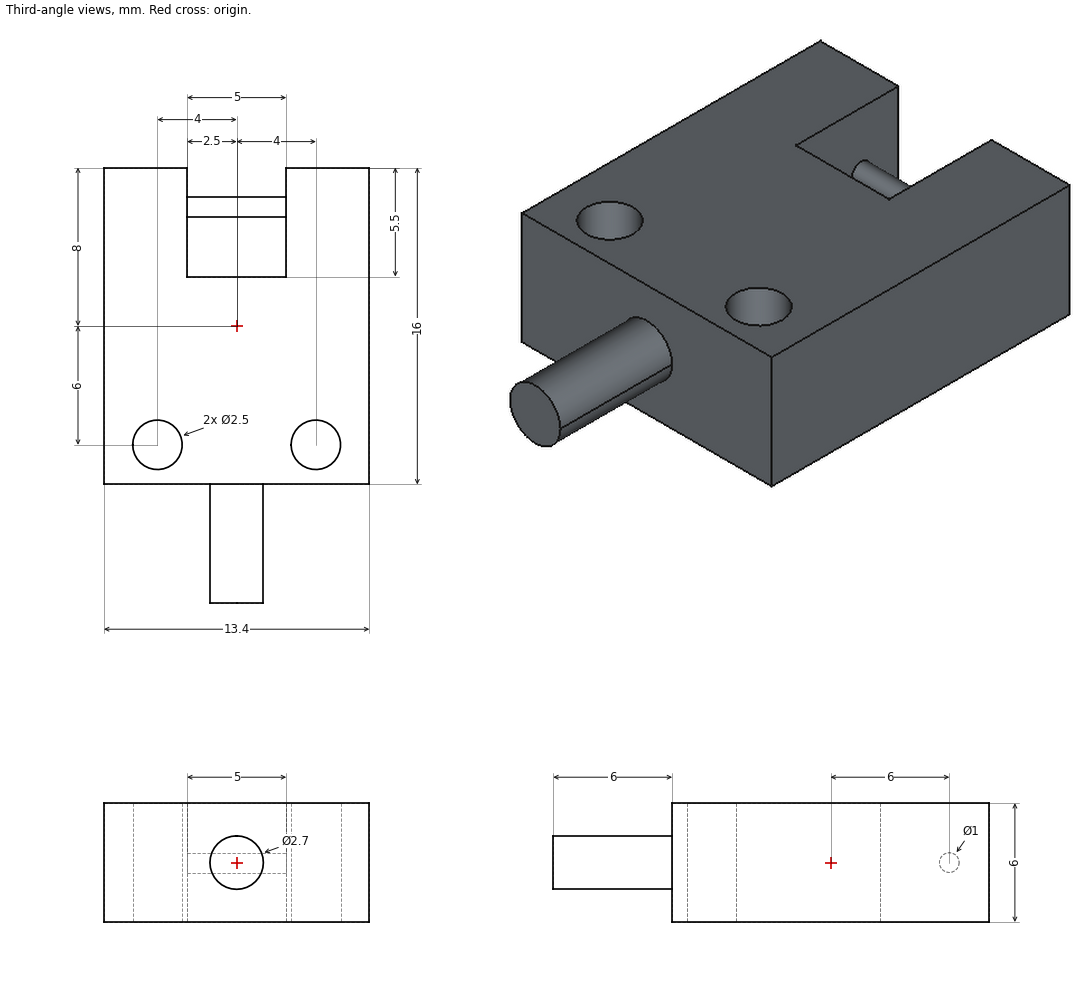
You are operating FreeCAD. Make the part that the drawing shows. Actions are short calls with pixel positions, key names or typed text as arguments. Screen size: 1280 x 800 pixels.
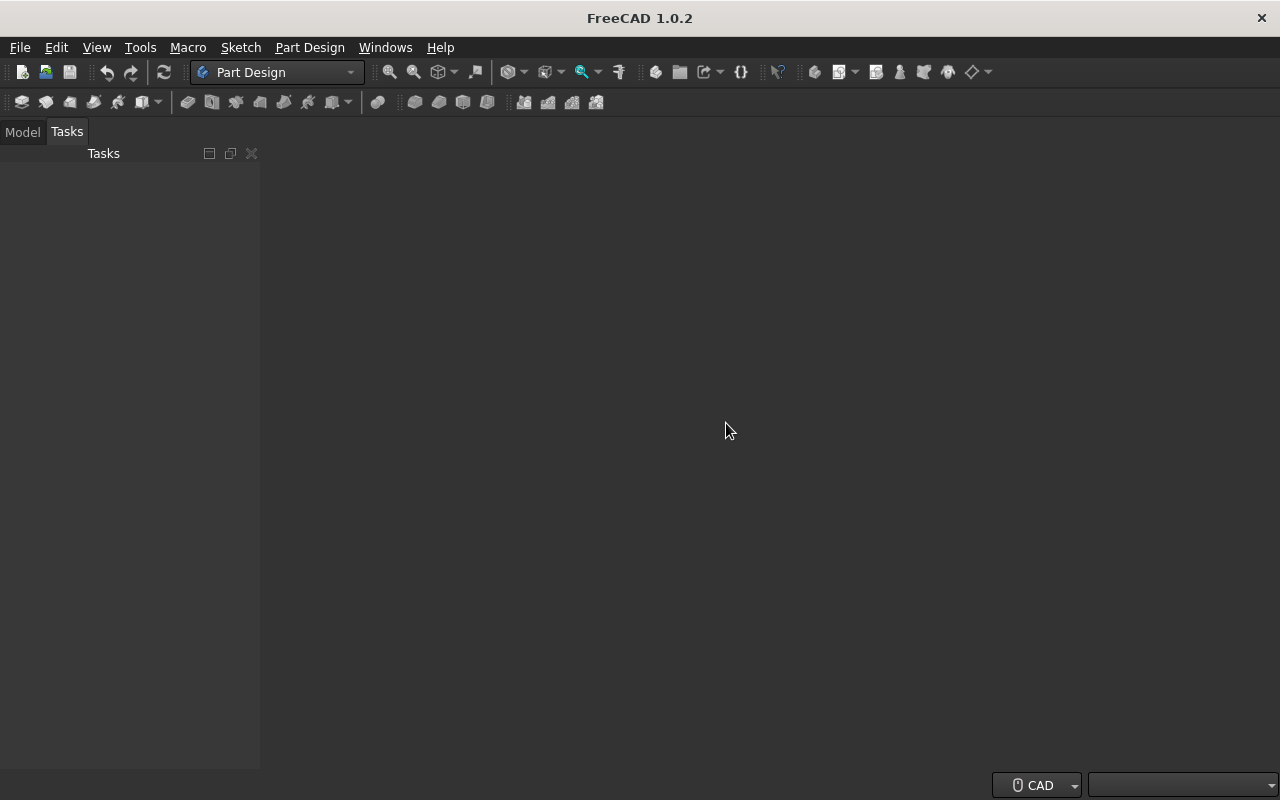
click(22, 72)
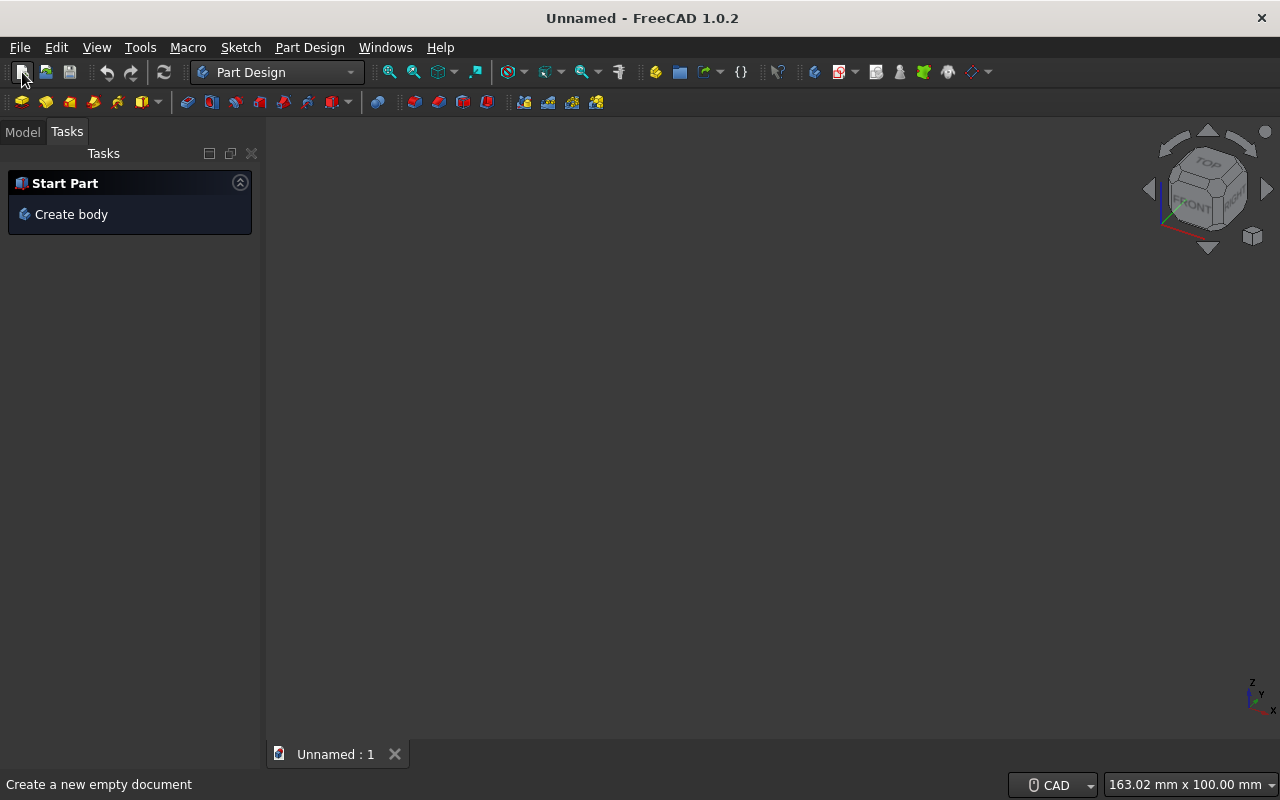
click(840, 72)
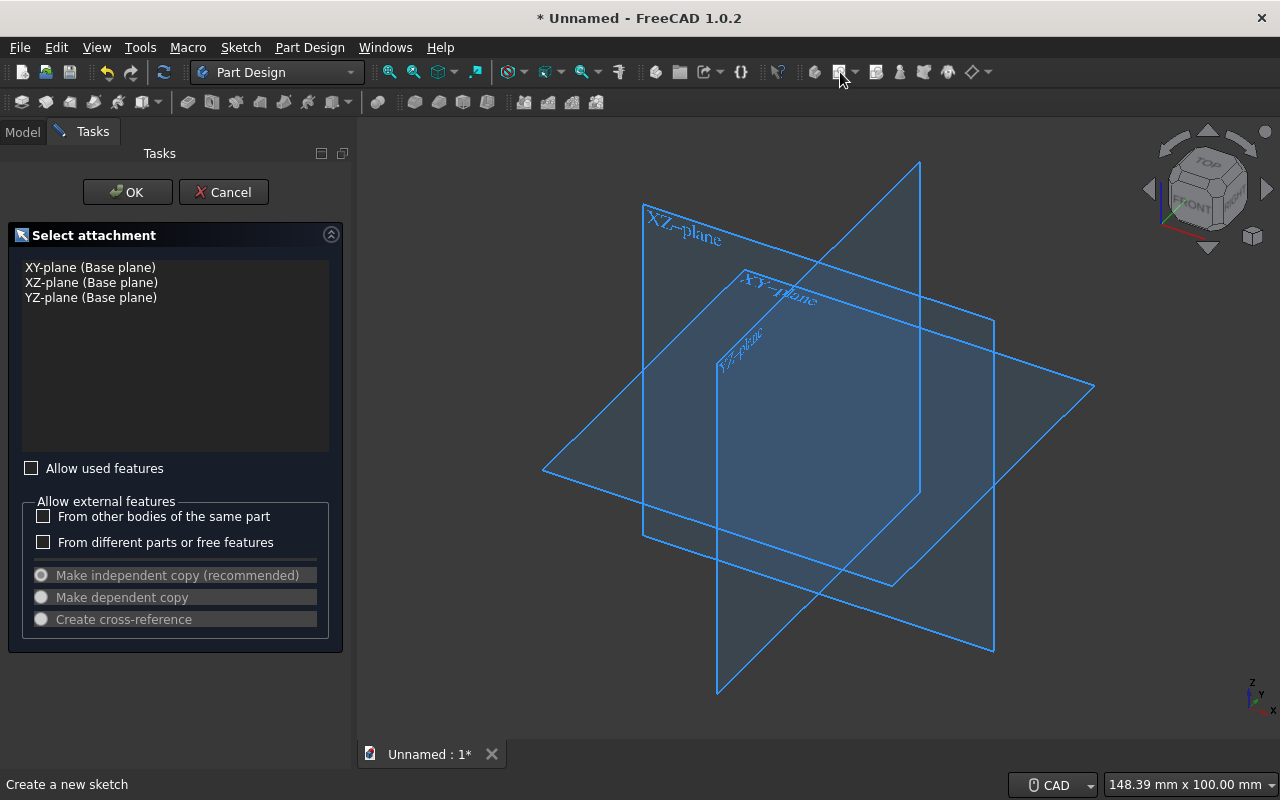
click(82, 268)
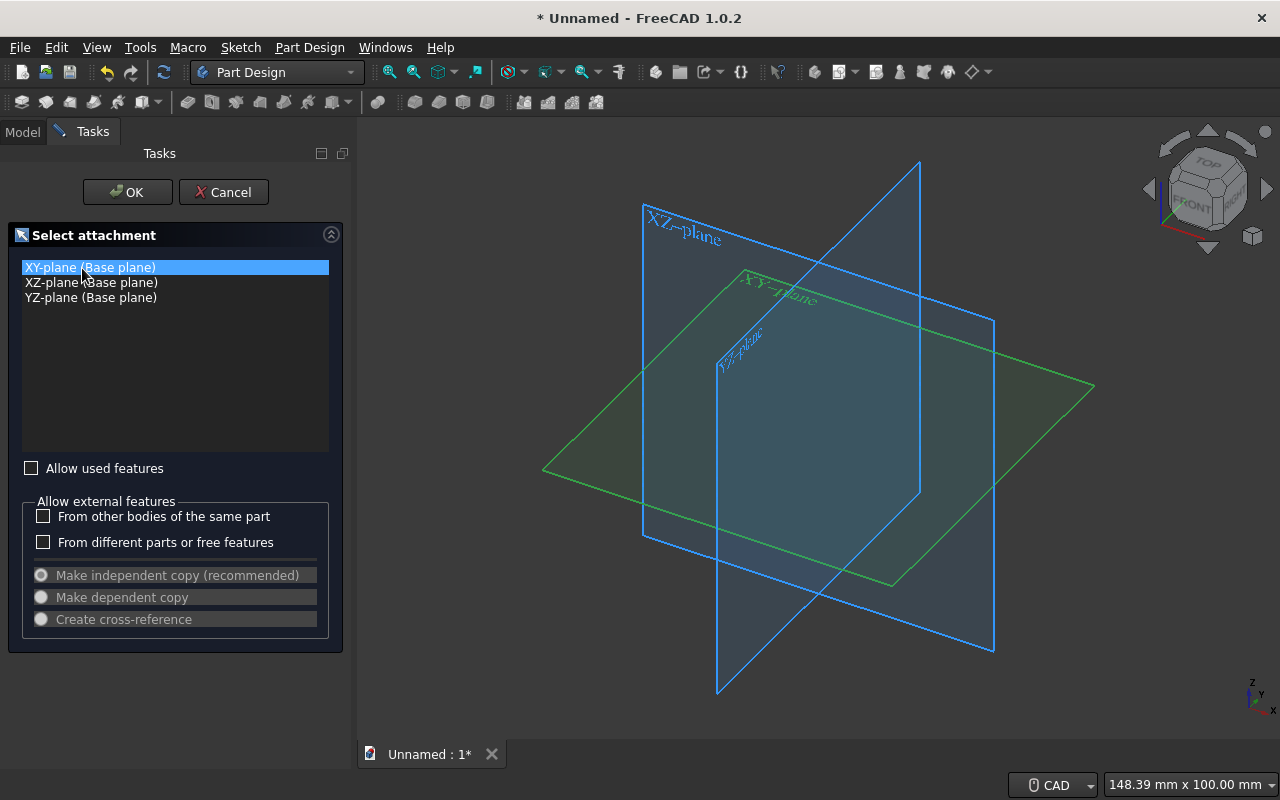
click(128, 192)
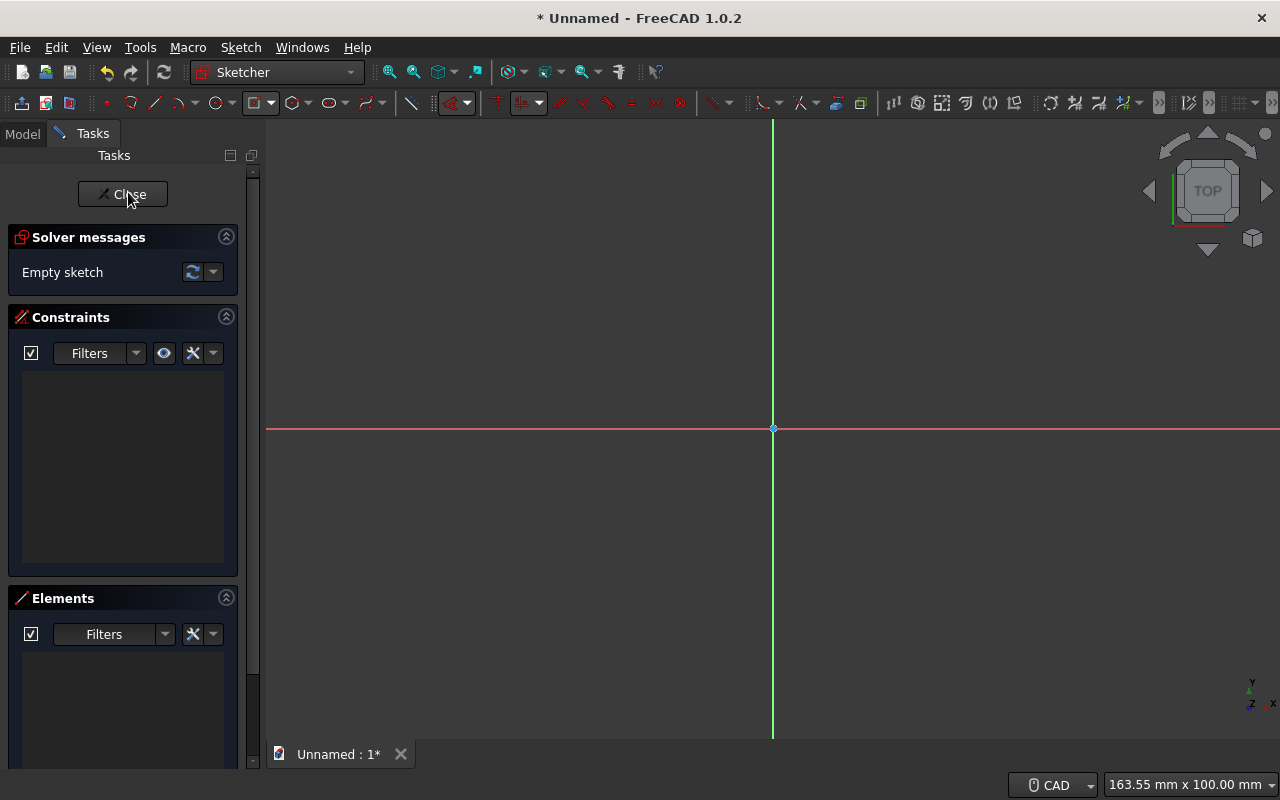
scroll(795, 429, up, 7)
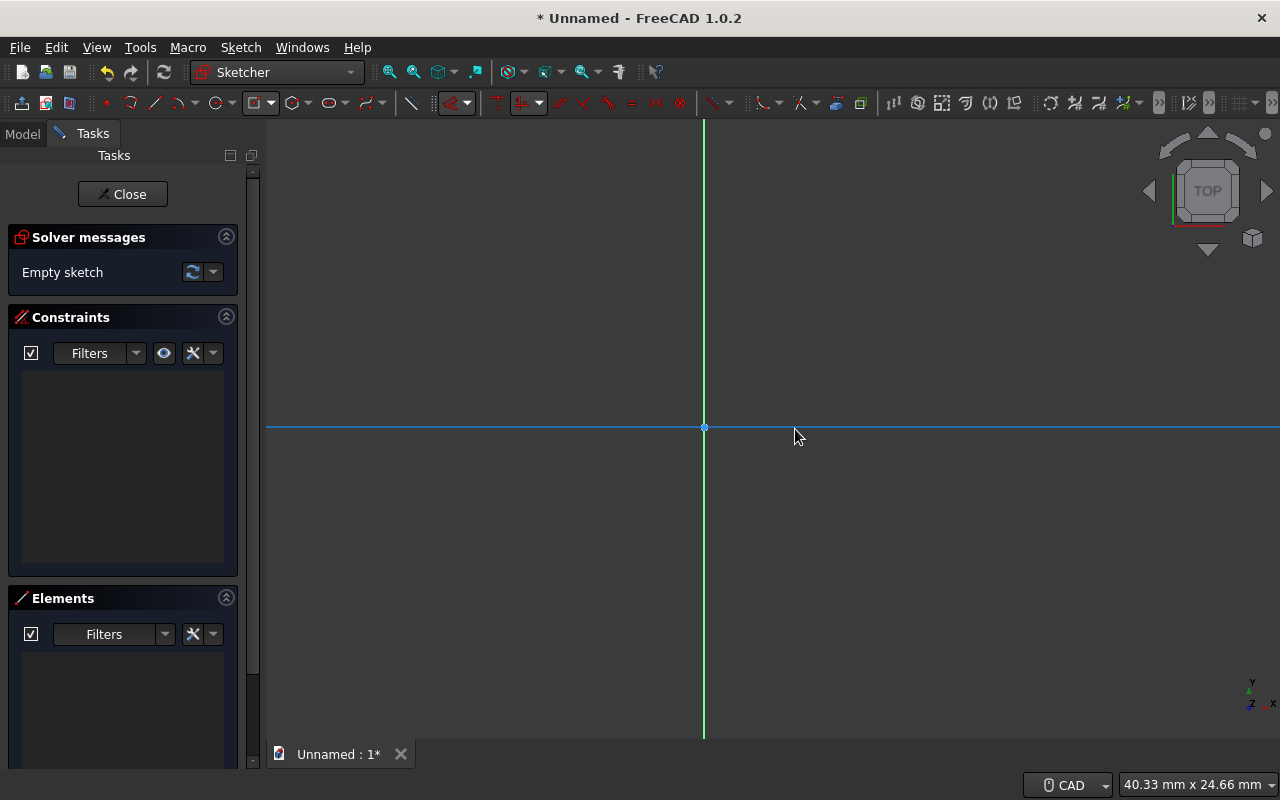
key(g)
key(v)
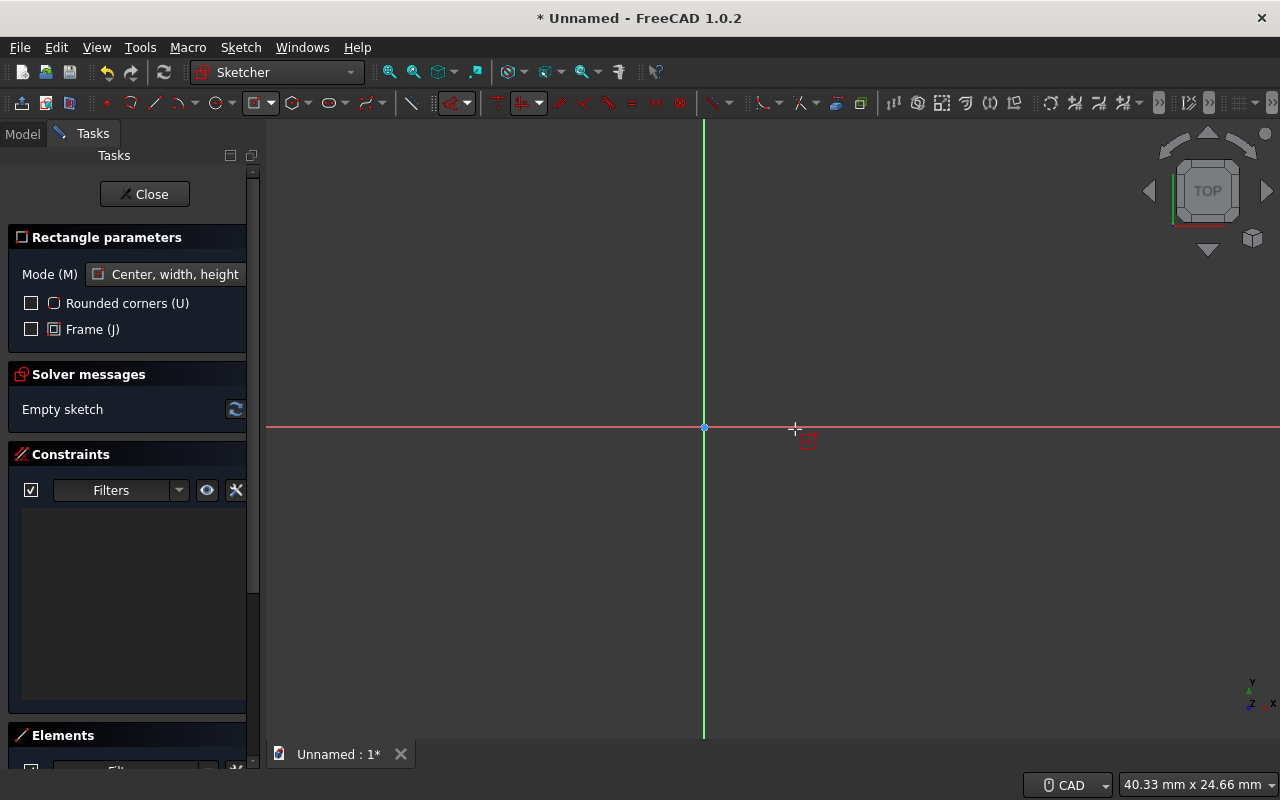
click(704, 427)
move(873, 226)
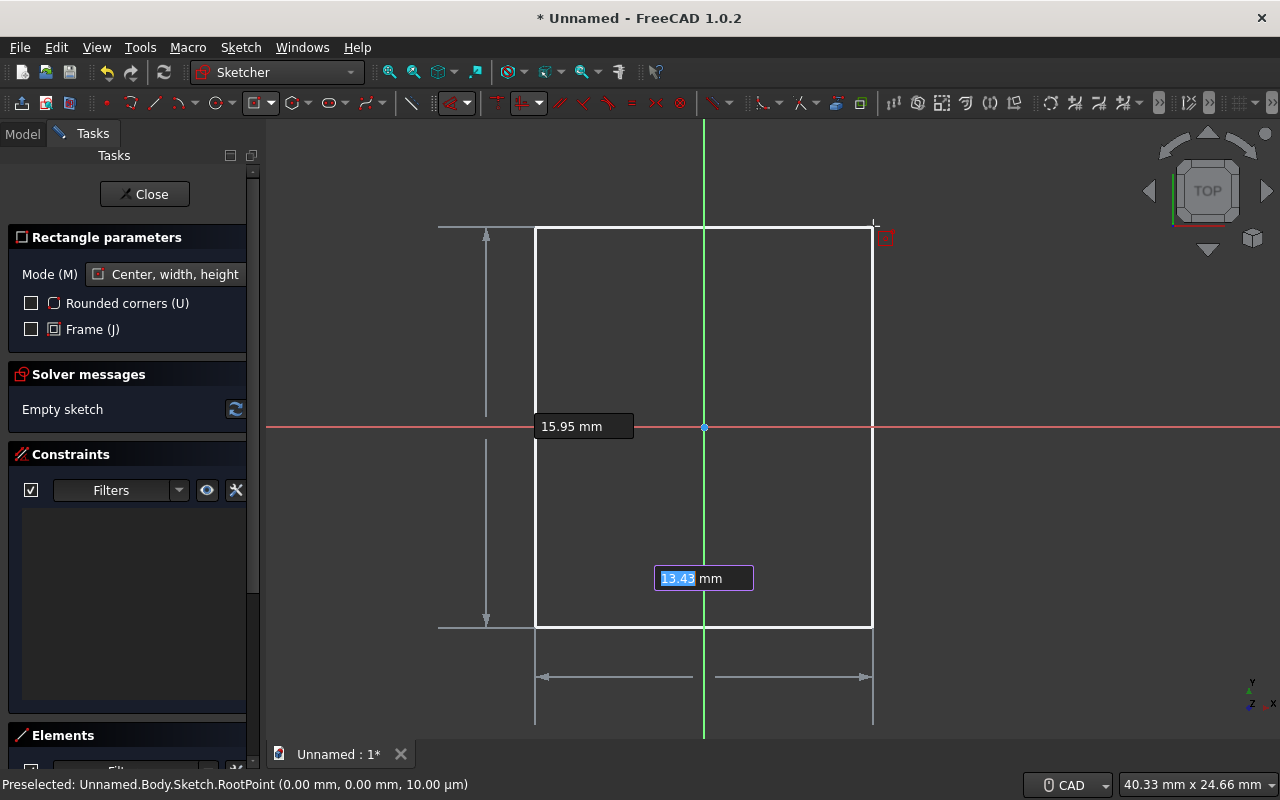
text(13.4)
key(Tab)
text(16)
key(Return)
key(Escape)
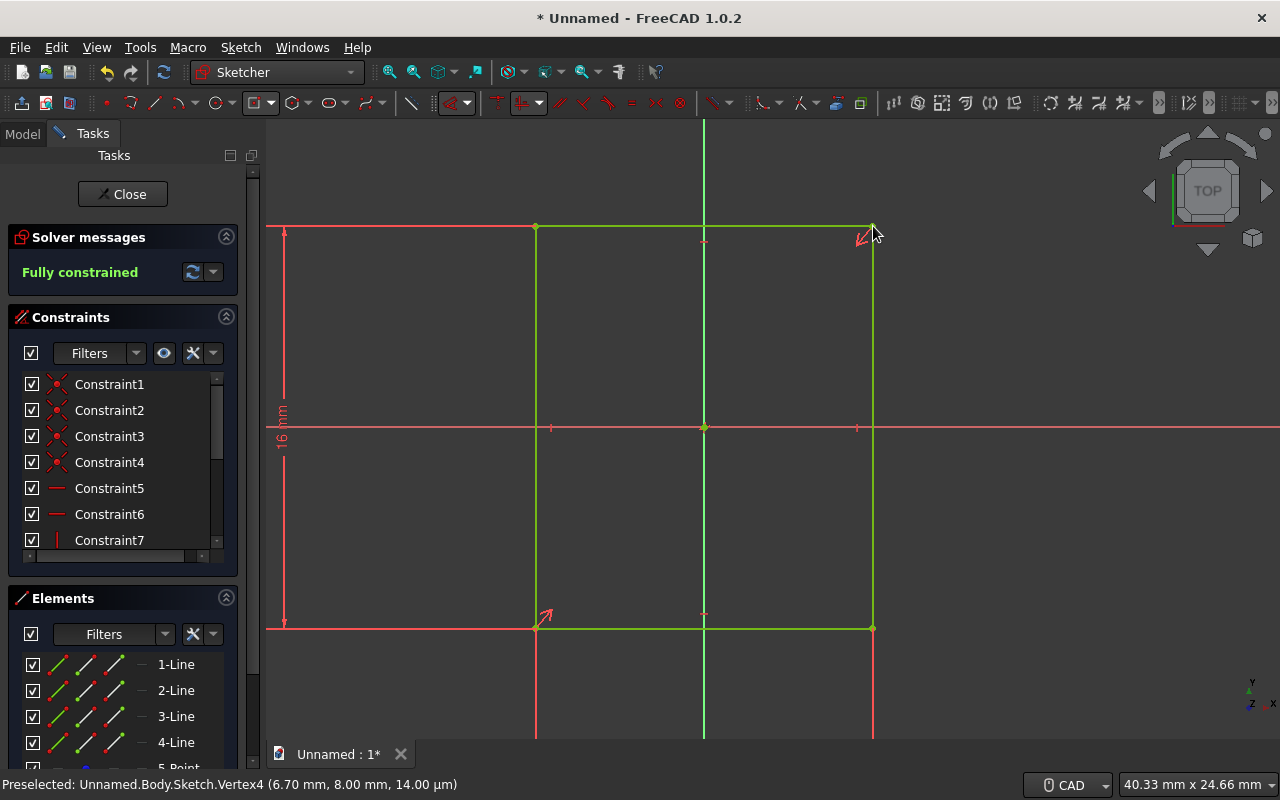
click(123, 194)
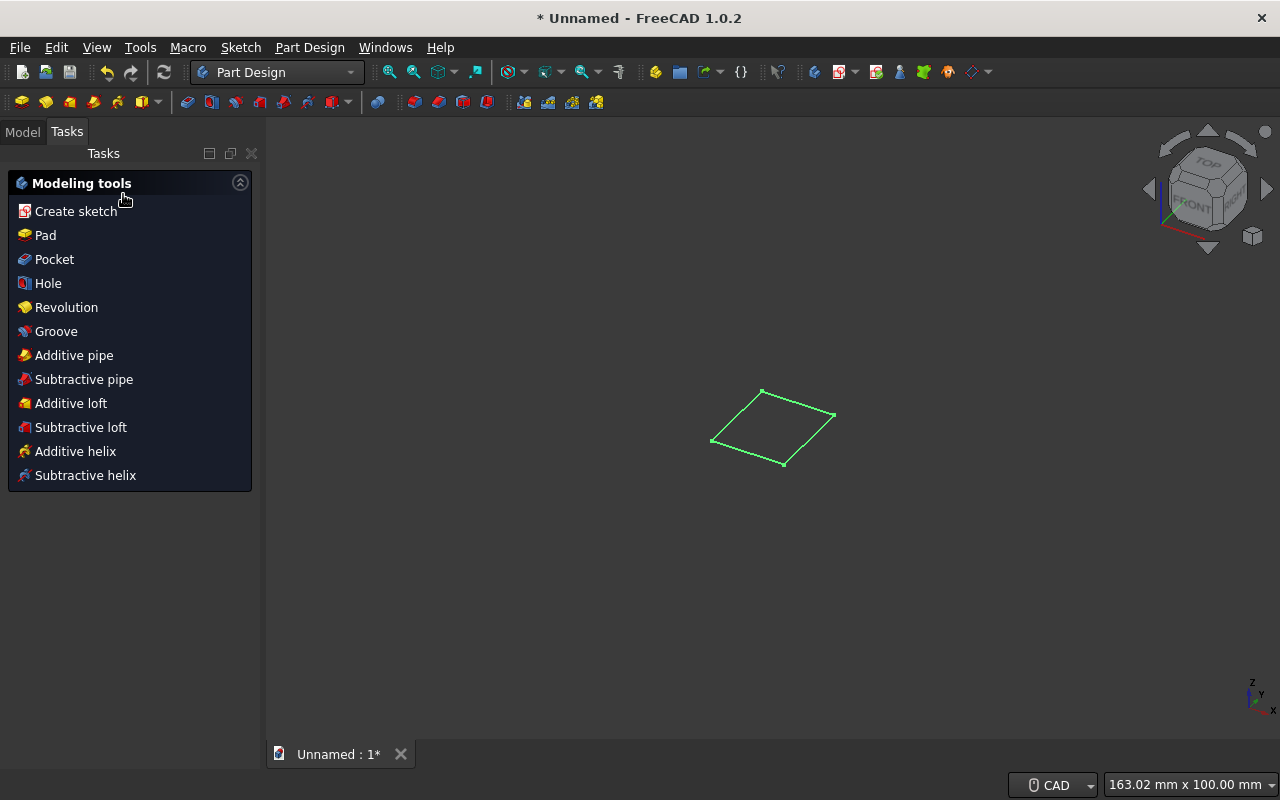
click(22, 102)